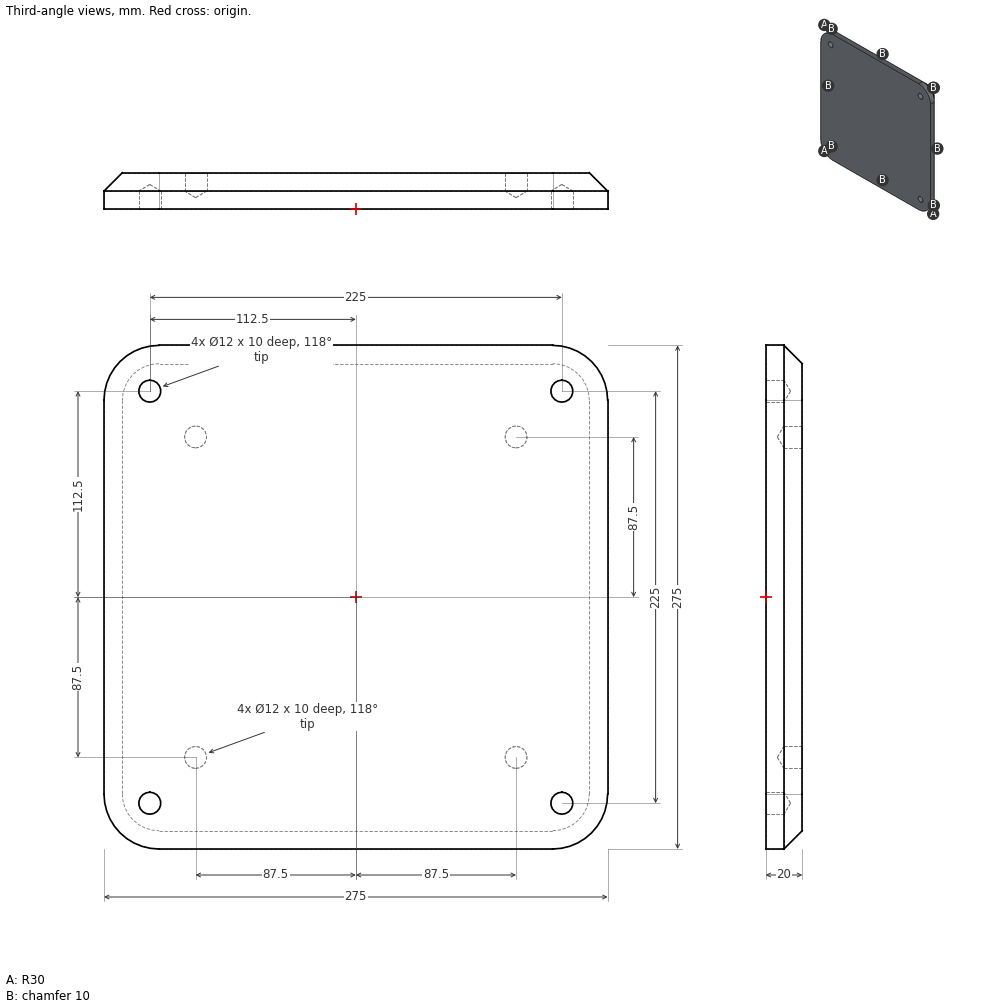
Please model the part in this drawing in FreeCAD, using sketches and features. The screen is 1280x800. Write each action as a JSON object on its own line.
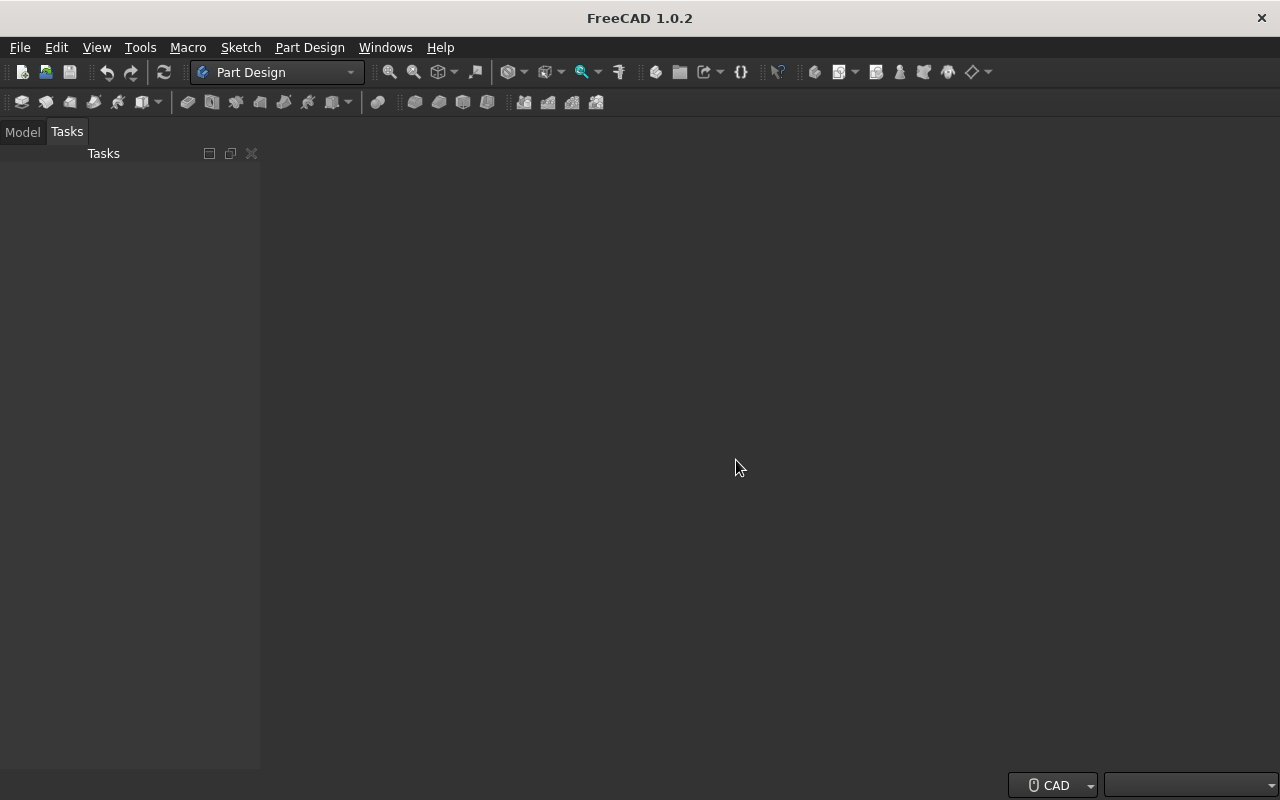
{"action": "left_click", "coordinate": [22, 72]}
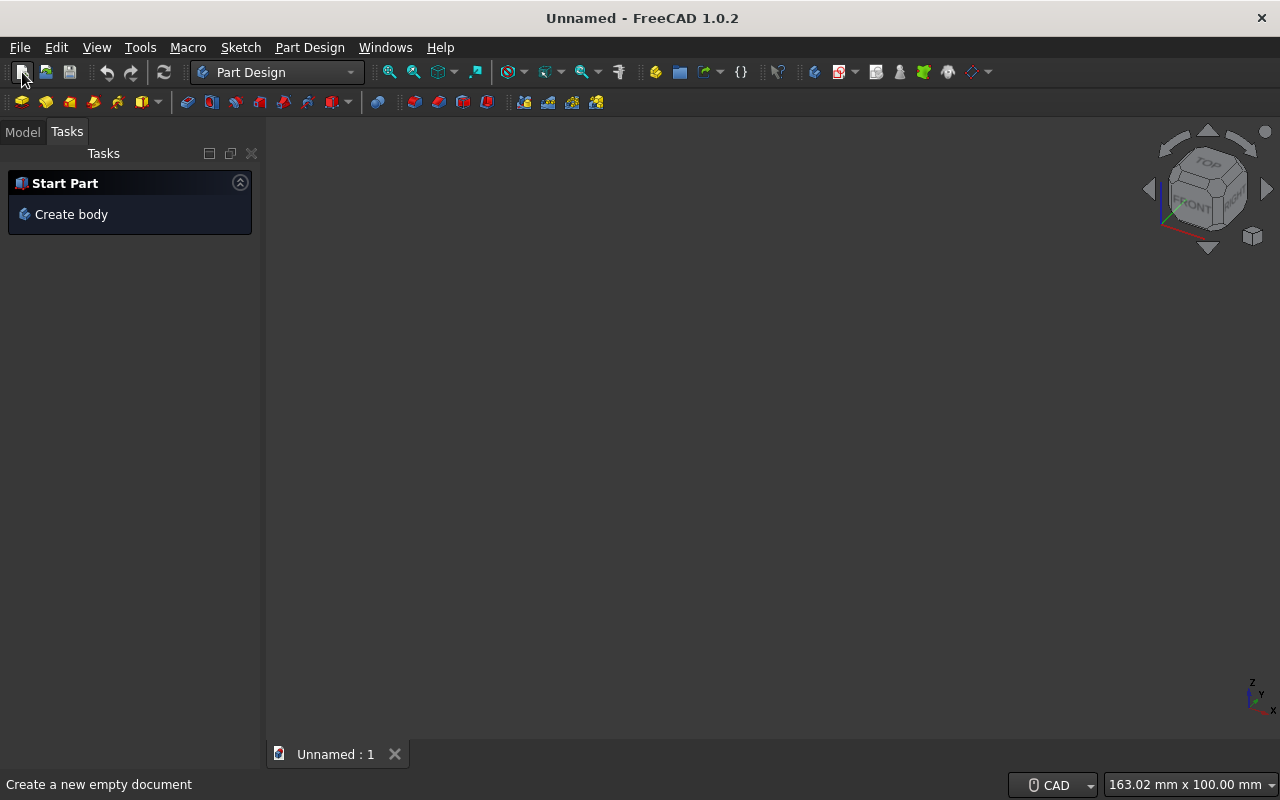
{"action": "left_click", "coordinate": [840, 72]}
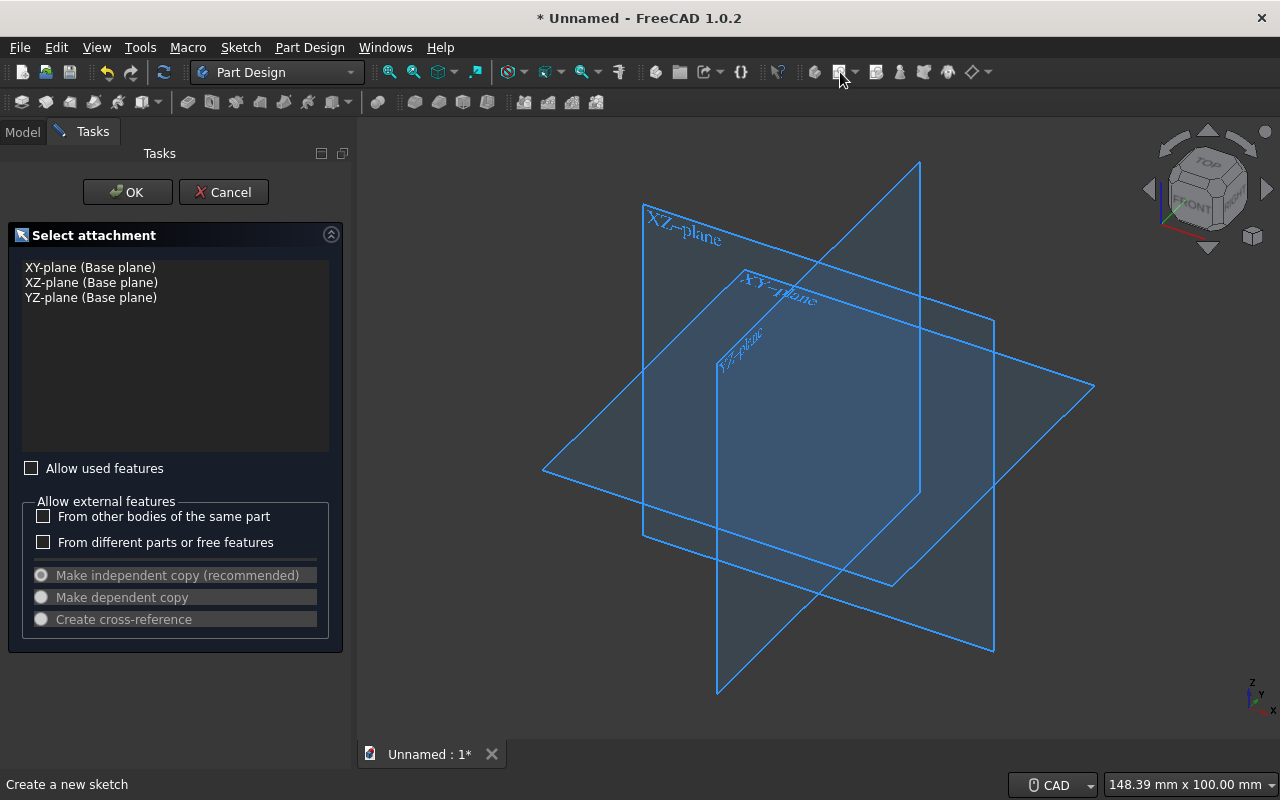
{"action": "left_click", "coordinate": [82, 282]}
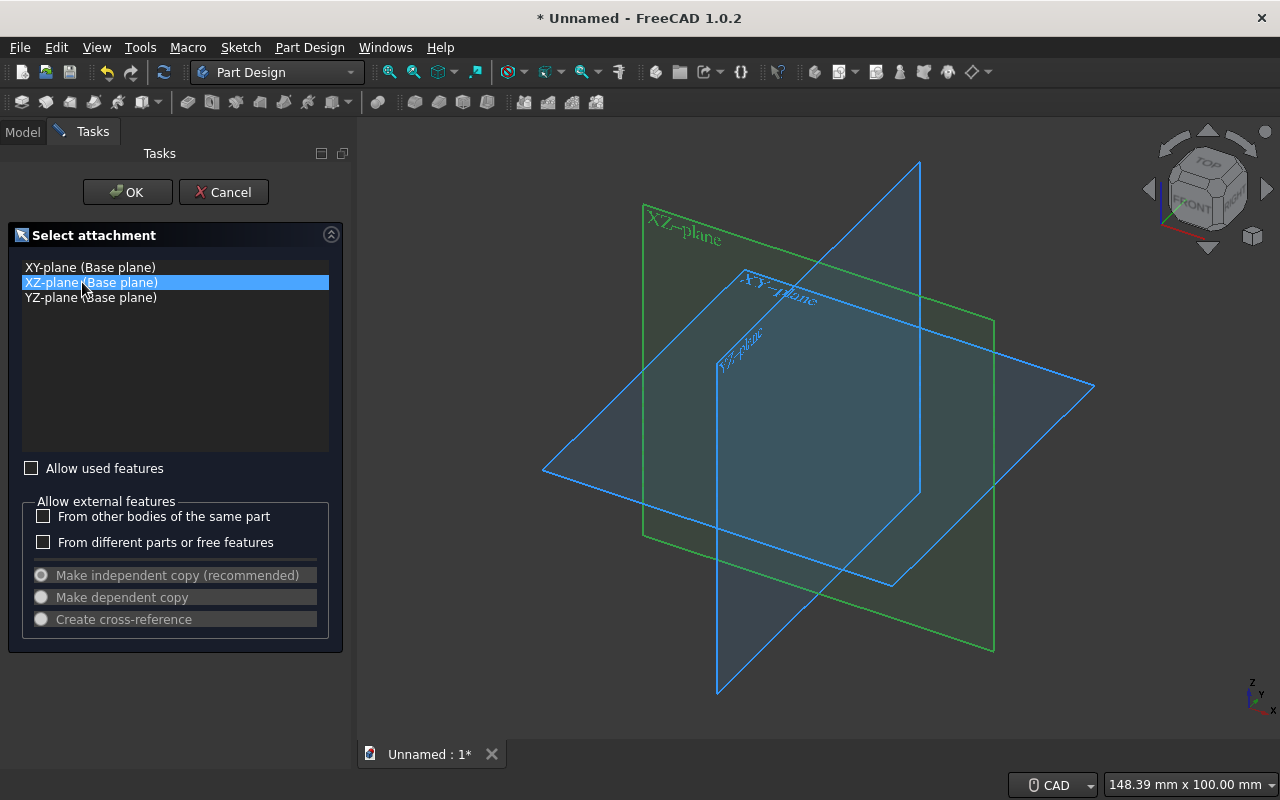
{"action": "left_click", "coordinate": [128, 192]}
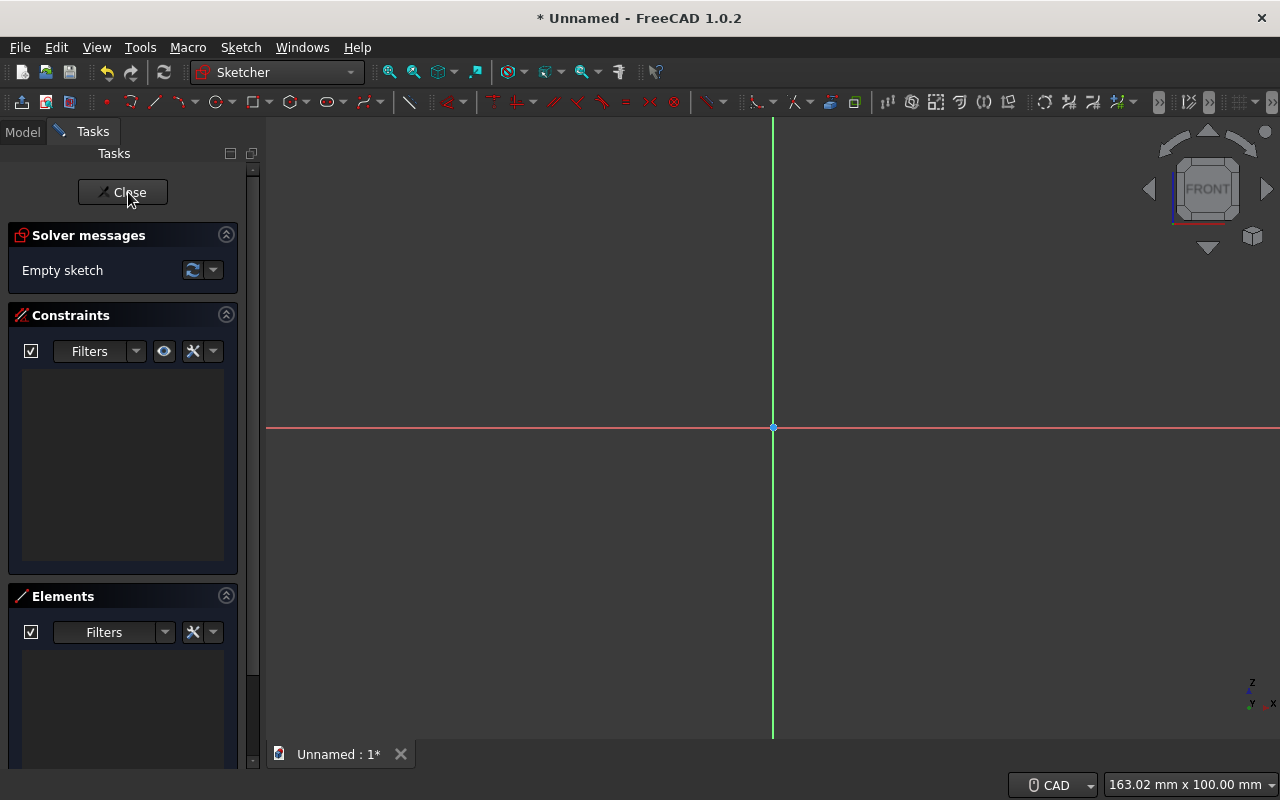
{"action": "scroll", "coordinate": [682, 428], "scroll_direction": "down", "scroll_amount": 7}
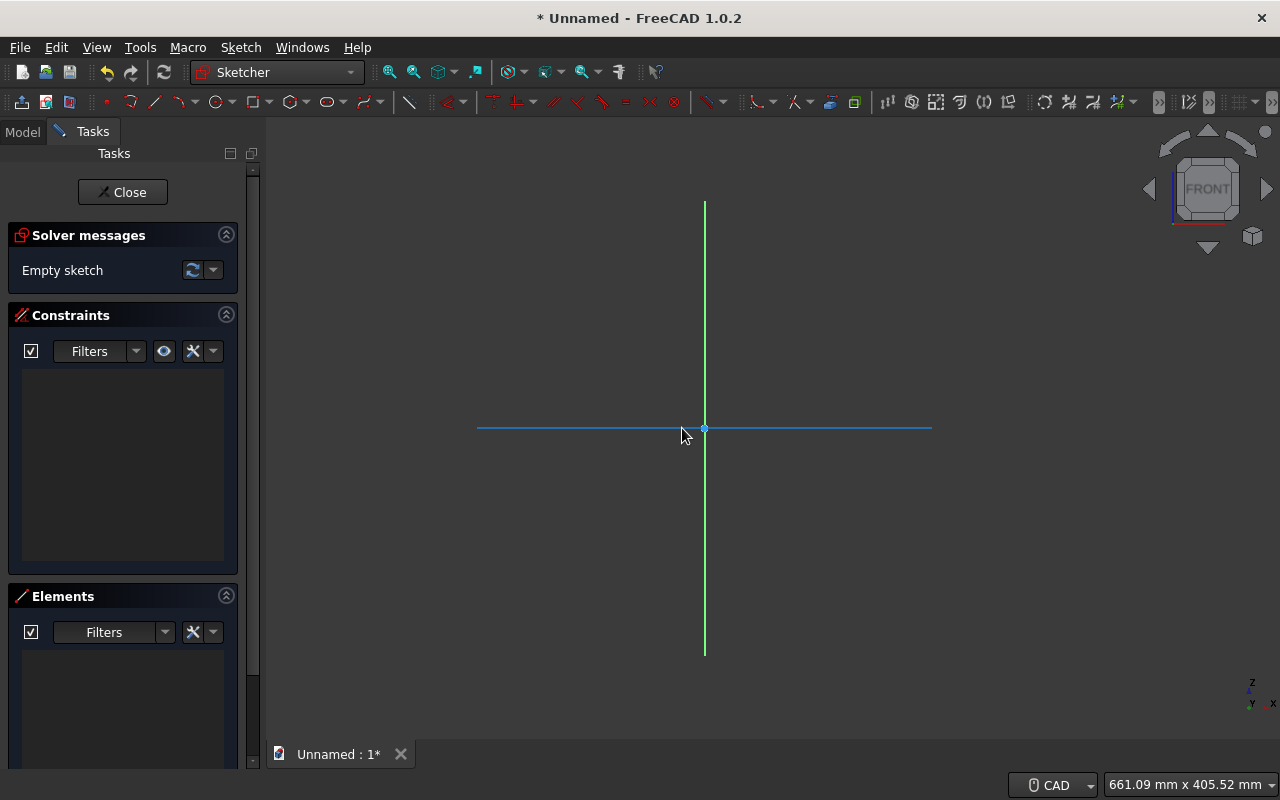
{"action": "key", "text": "g v"}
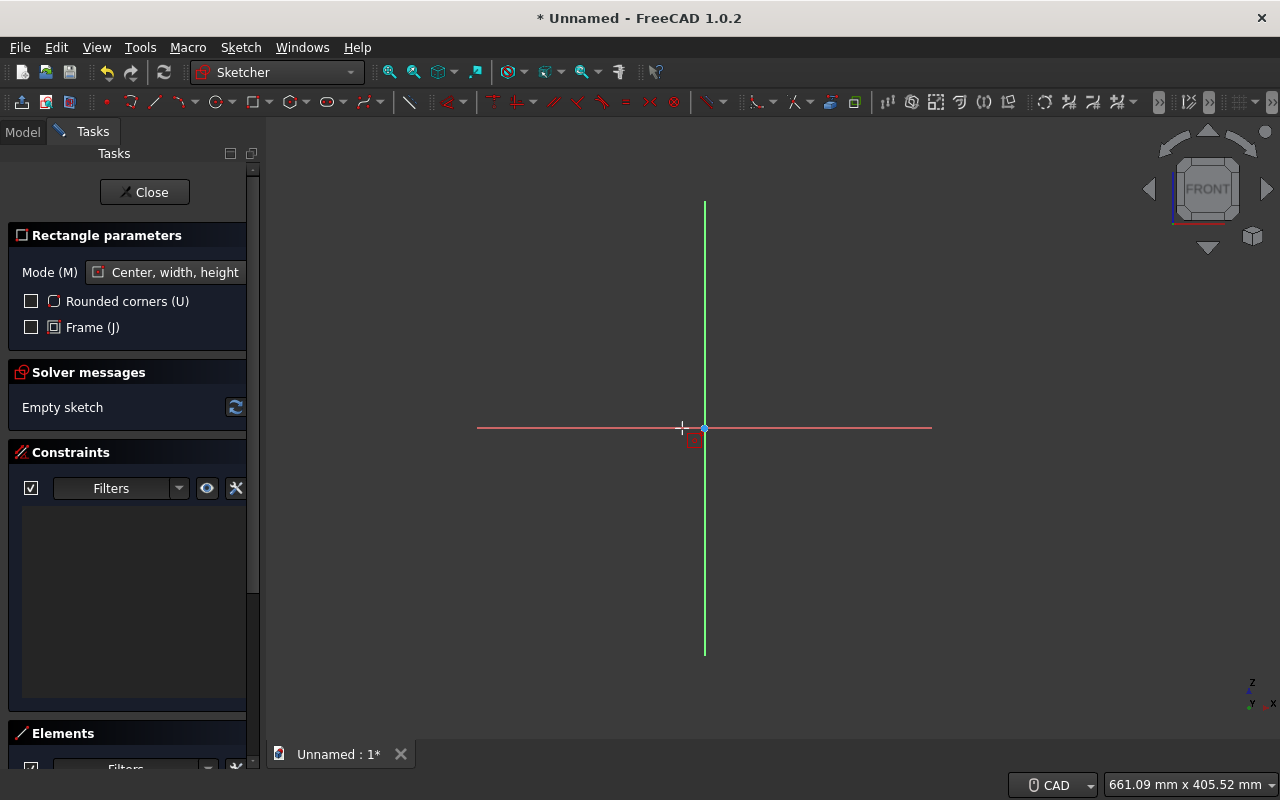
{"action": "left_click", "coordinate": [705, 428]}
{"action": "mouse_move", "coordinate": [916, 217]}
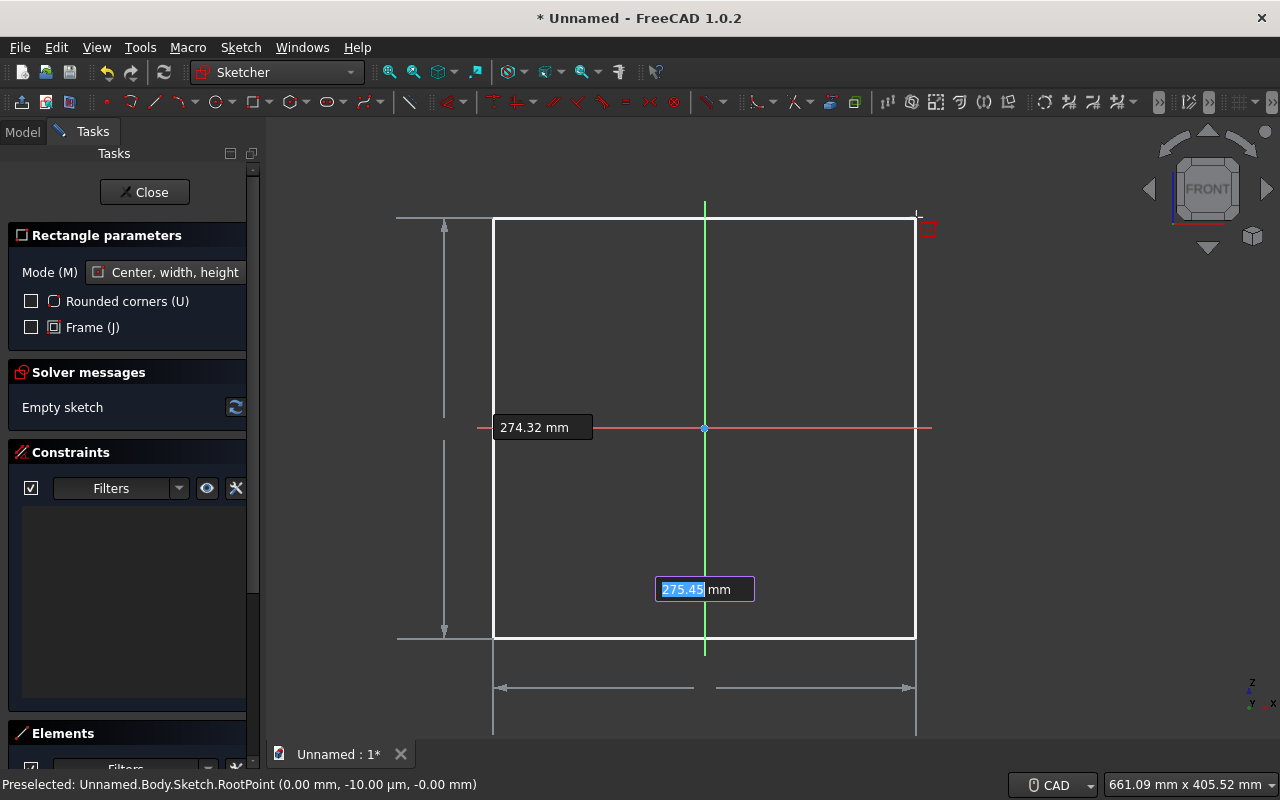
{"action": "type", "text": "275"}
{"action": "key", "text": "Tab"}
{"action": "type", "text": "275"}
{"action": "key", "text": "Return"}
{"action": "key", "text": "Escape"}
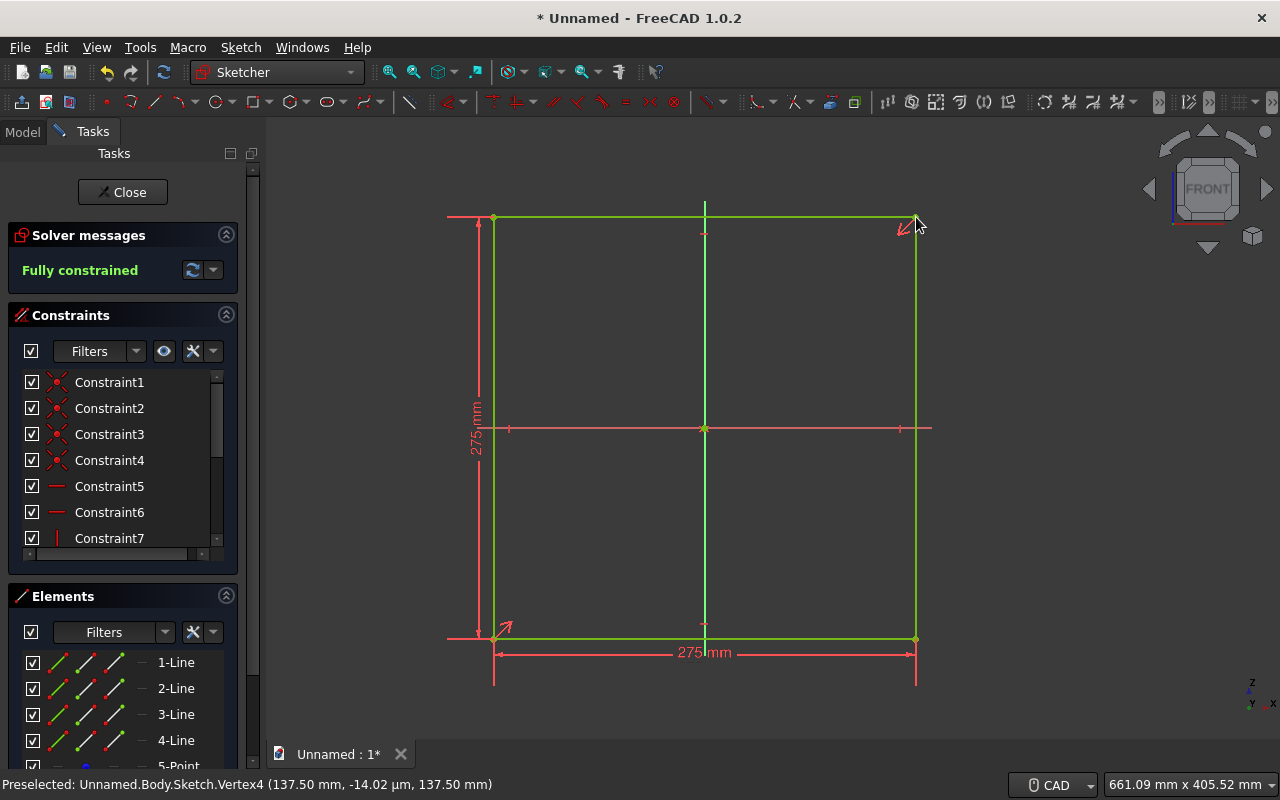
{"action": "left_click", "coordinate": [123, 192]}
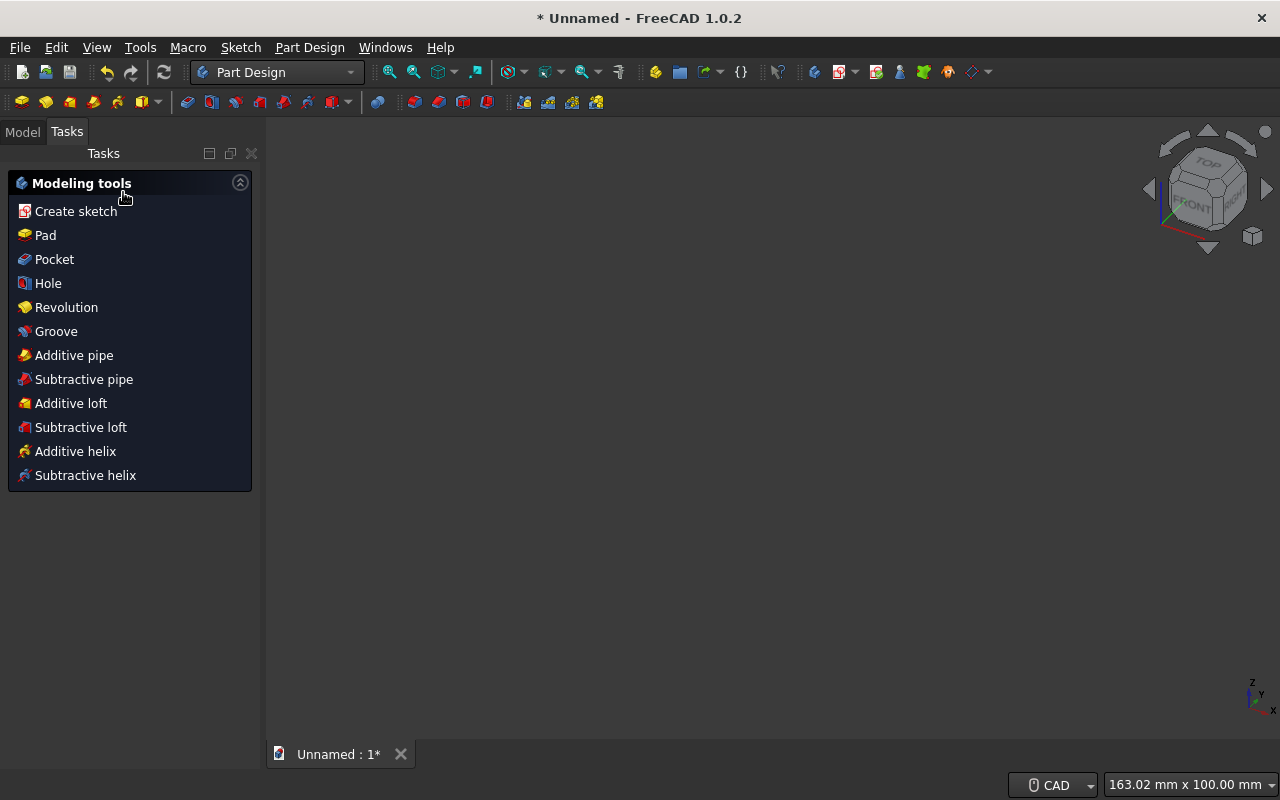
{"action": "left_click", "coordinate": [22, 102]}